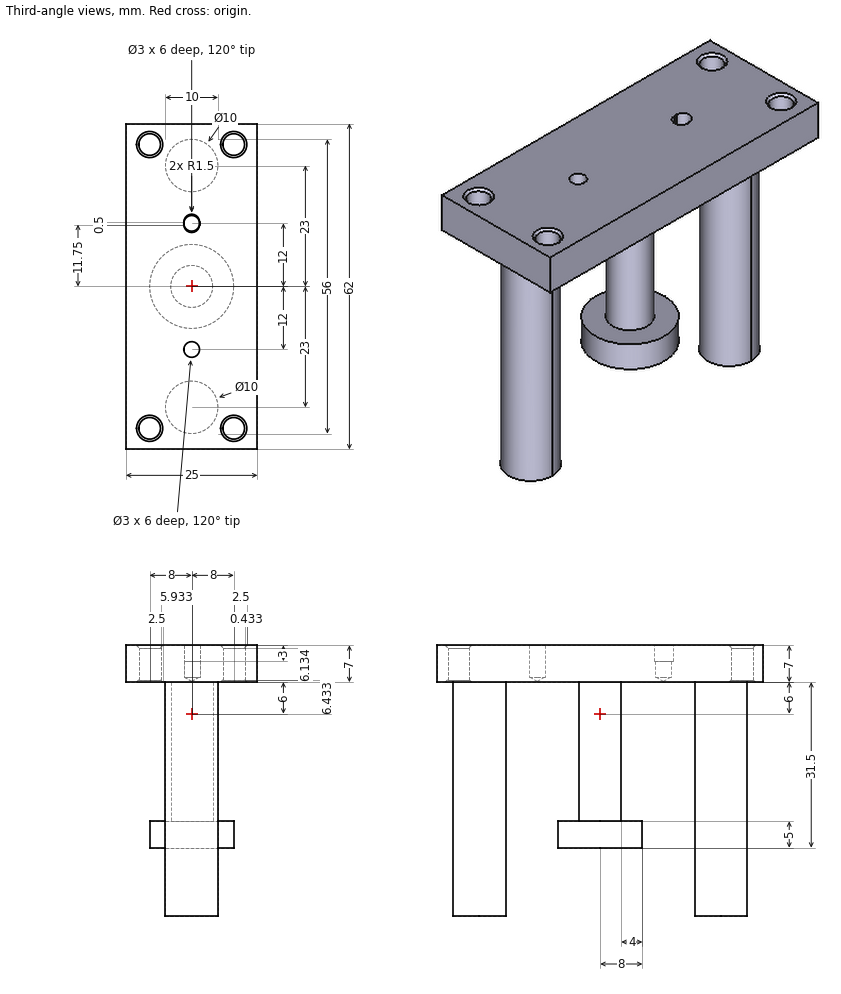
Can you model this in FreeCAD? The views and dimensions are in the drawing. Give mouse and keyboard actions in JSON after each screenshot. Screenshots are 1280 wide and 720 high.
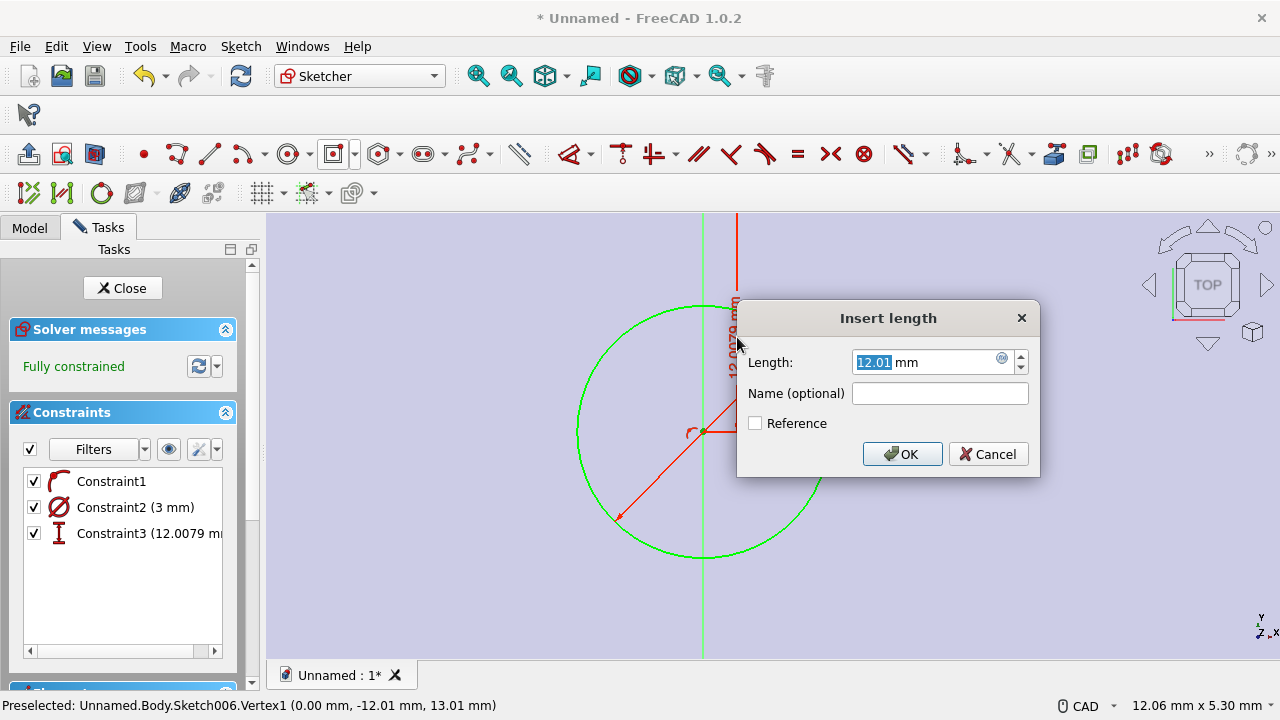
{"action": "type", "text": "12"}
{"action": "key", "text": "Return"}
{"action": "key", "text": "Escape"}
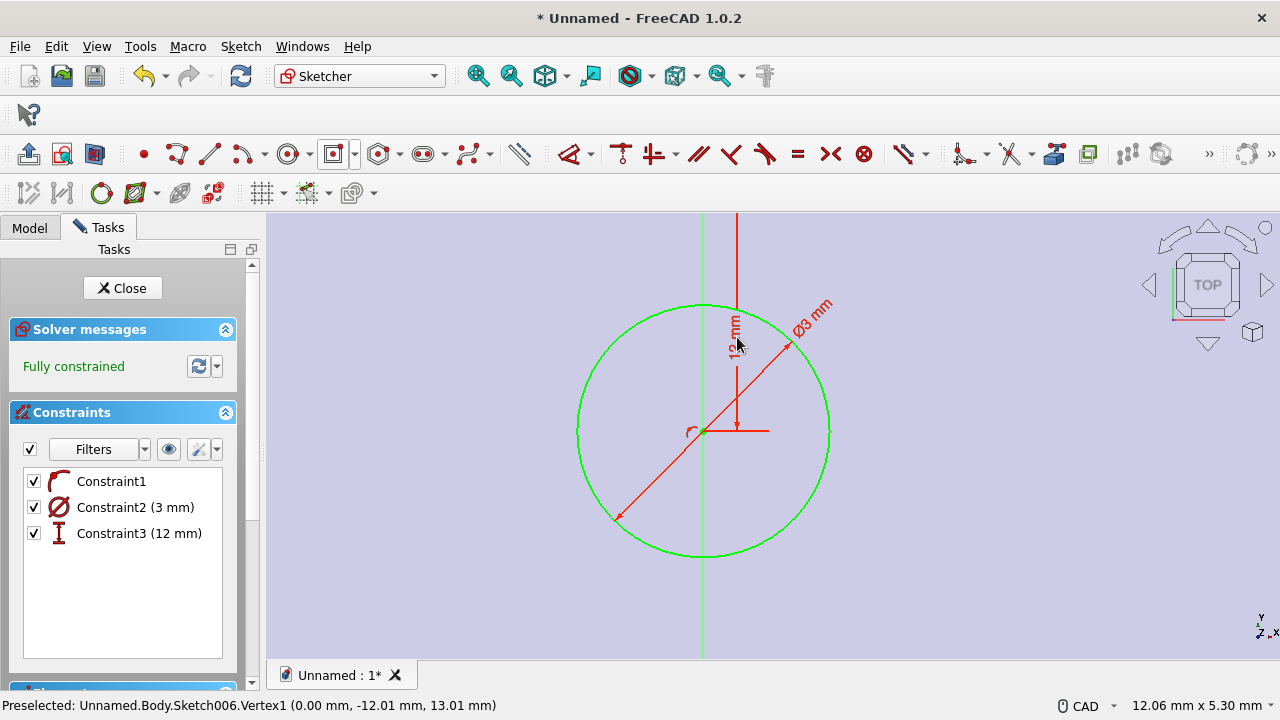
{"action": "left_click", "coordinate": [123, 288]}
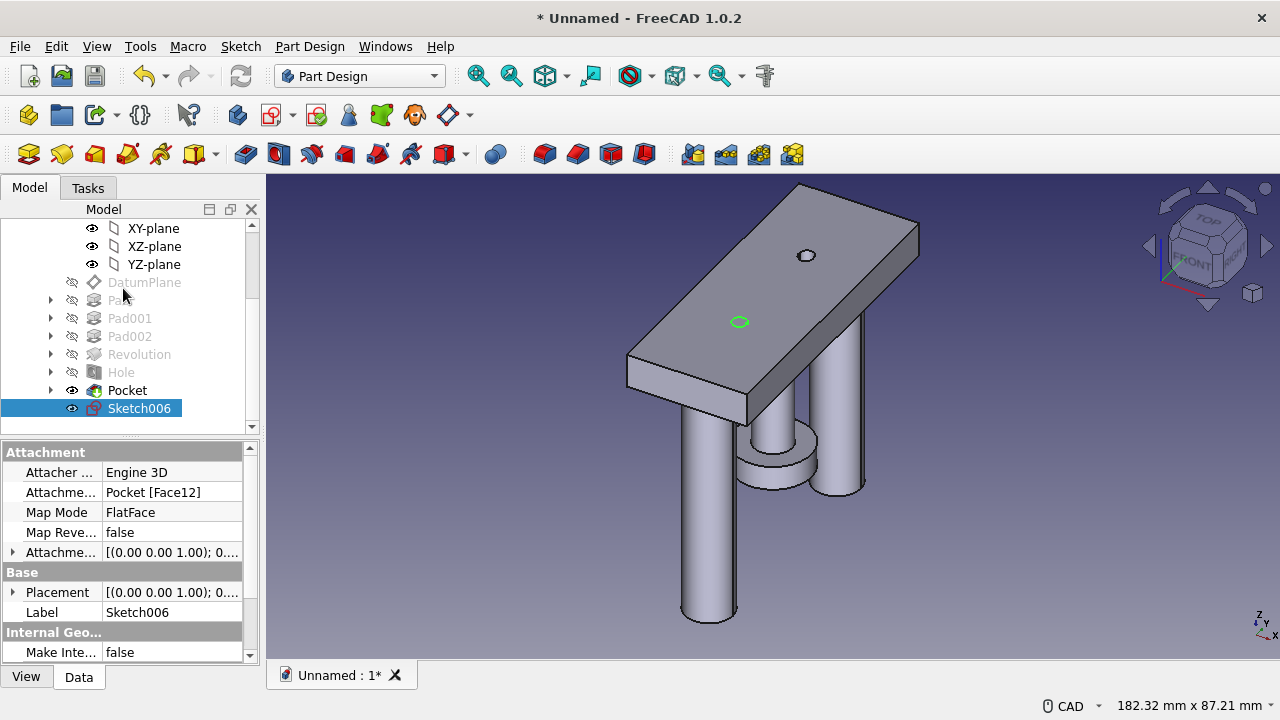
{"action": "left_click", "coordinate": [279, 154]}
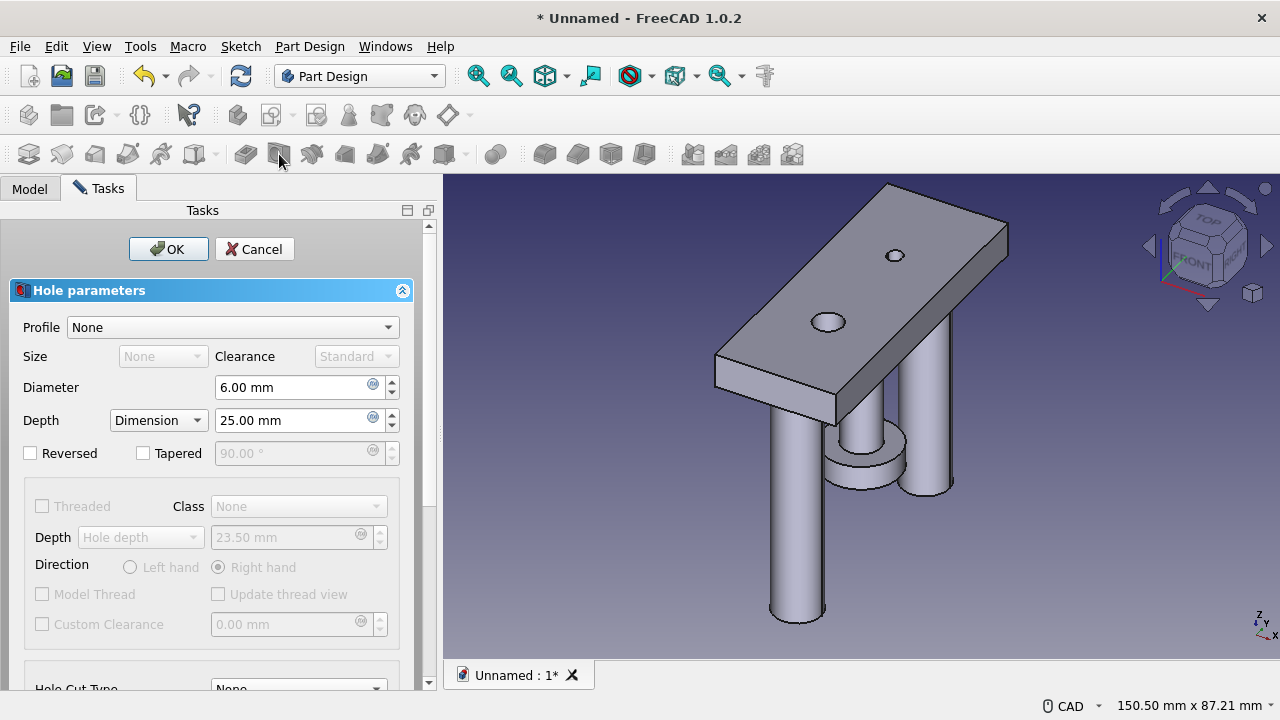
{"action": "triple_click", "coordinate": [300, 388]}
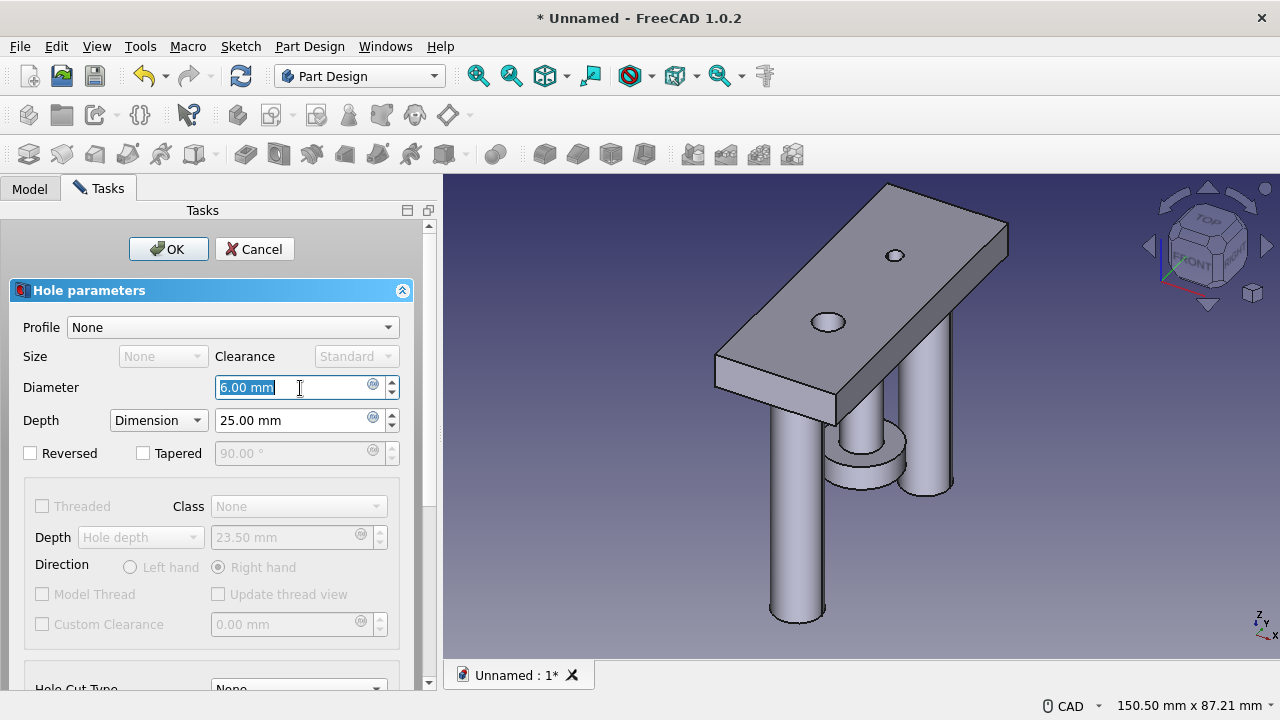
{"action": "type", "text": "3"}
{"action": "key", "text": "Tab"}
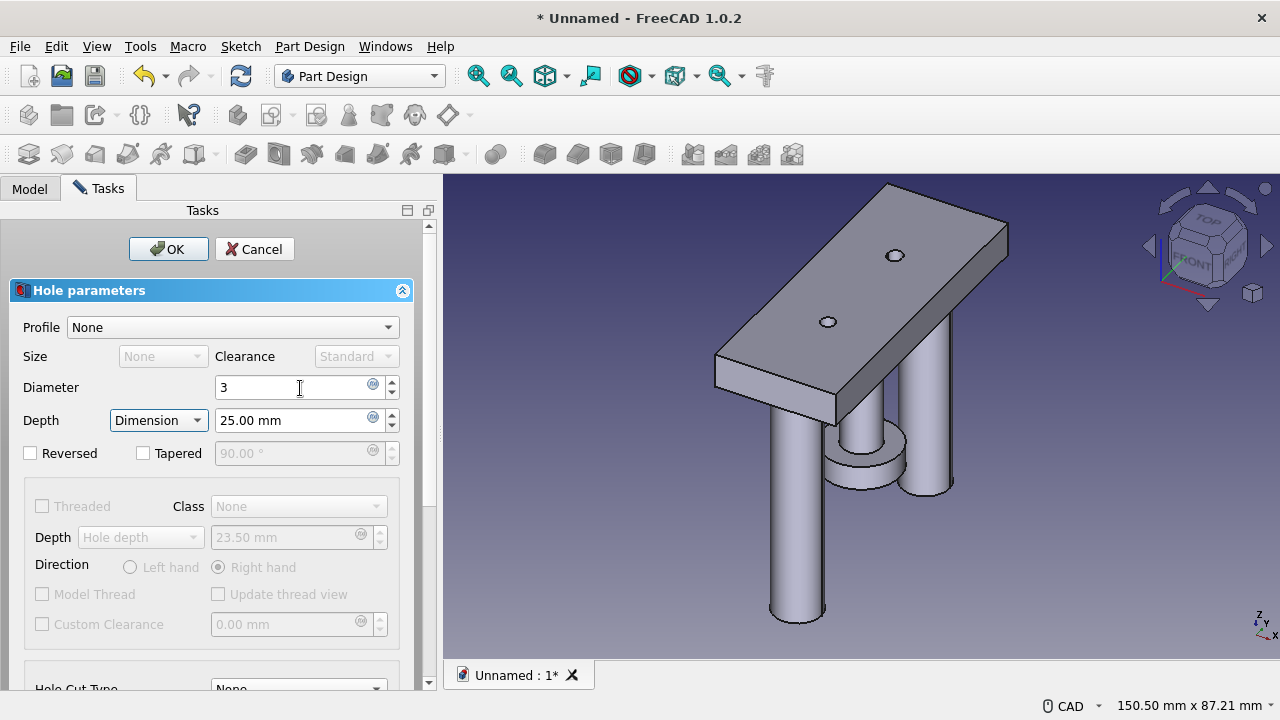
{"action": "triple_click", "coordinate": [300, 420]}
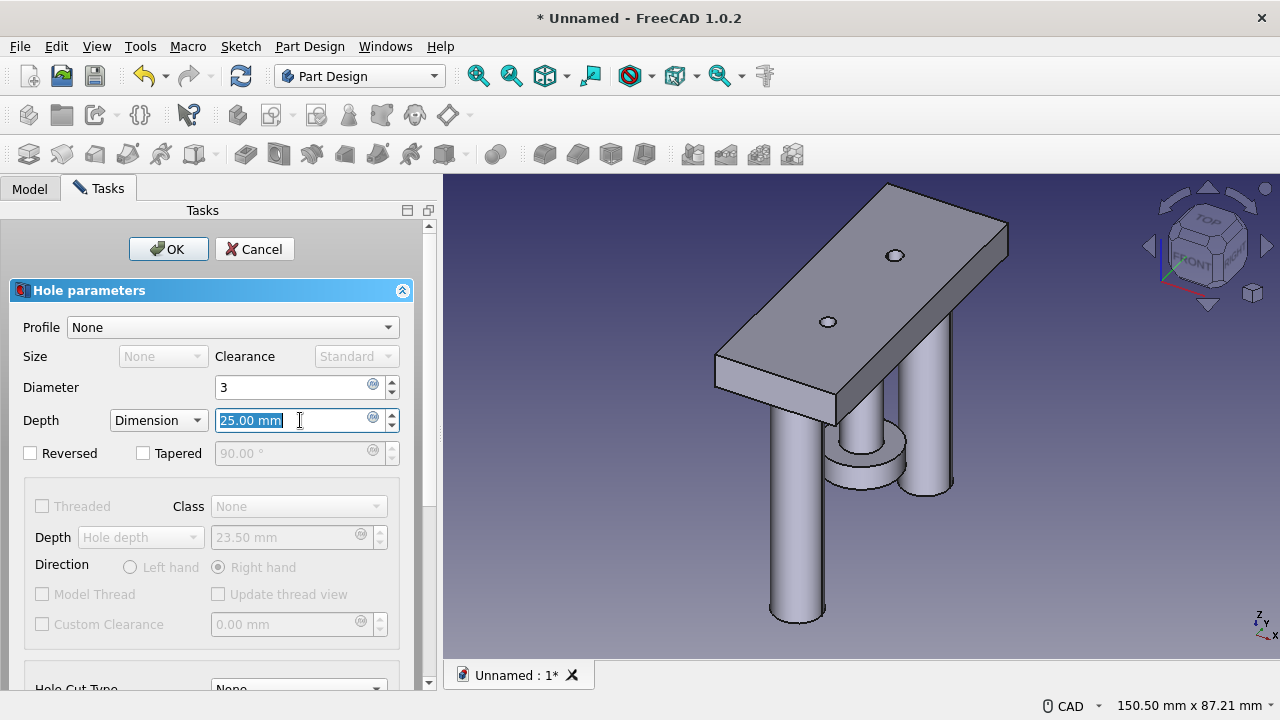
{"action": "type", "text": "6"}
{"action": "key", "text": "Tab"}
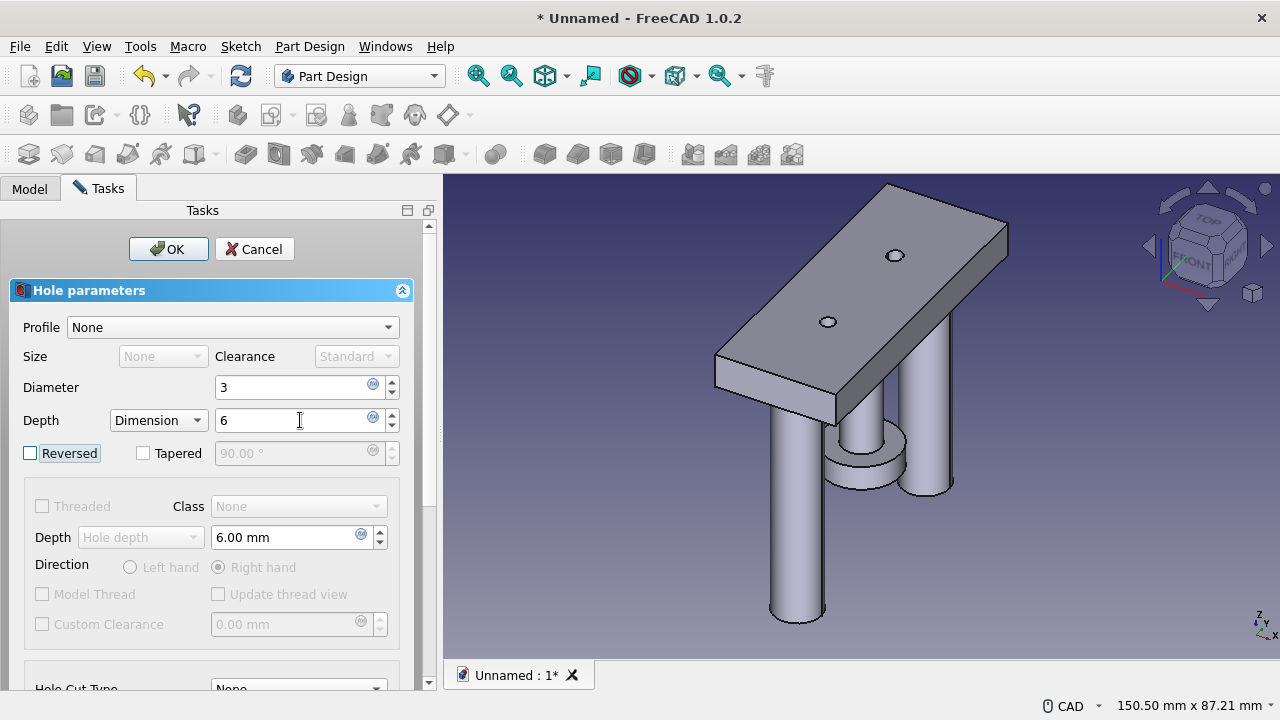
{"action": "scroll", "coordinate": [429, 455], "scroll_direction": "down", "scroll_amount": 5}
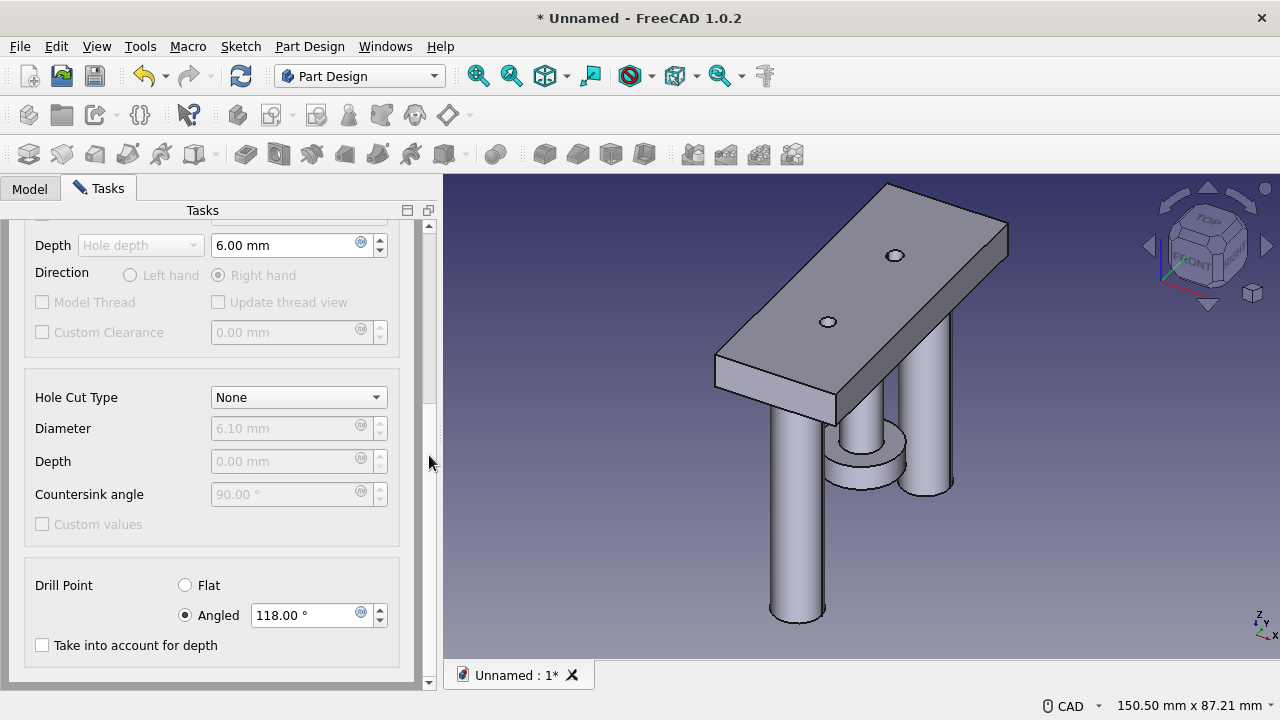
{"action": "triple_click", "coordinate": [312, 616]}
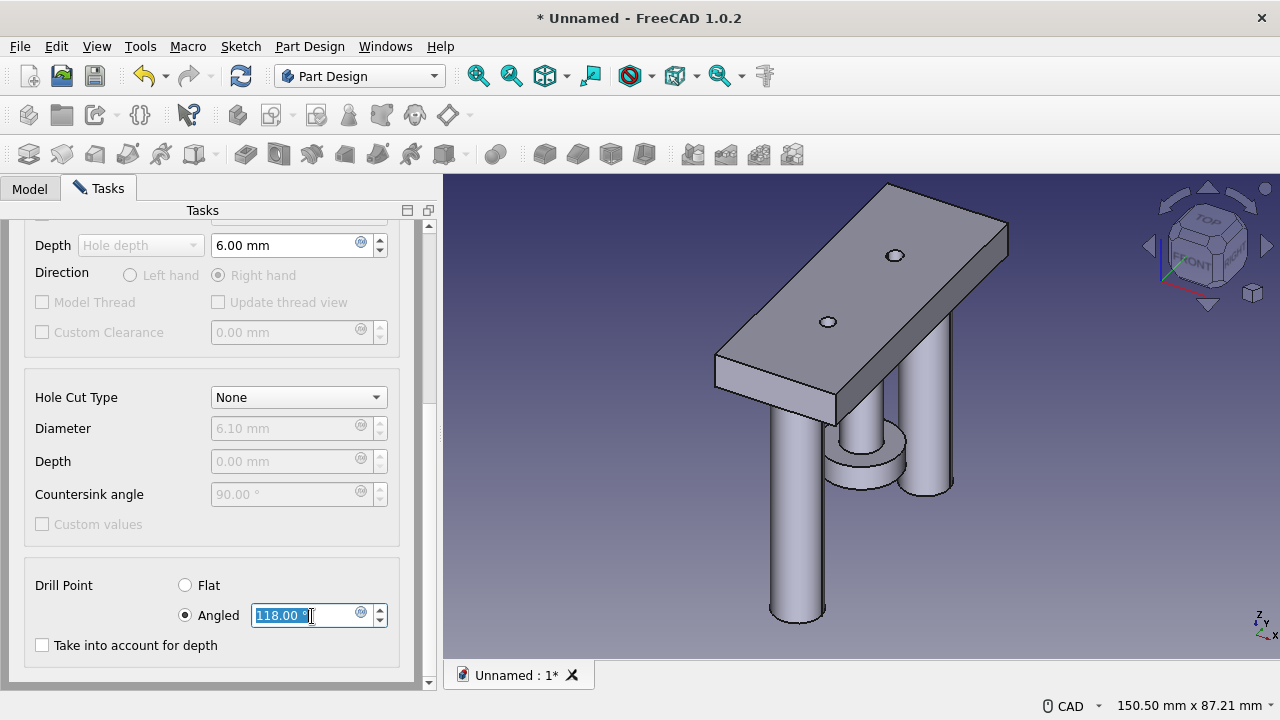
{"action": "type", "text": "120"}
{"action": "key", "text": "Tab"}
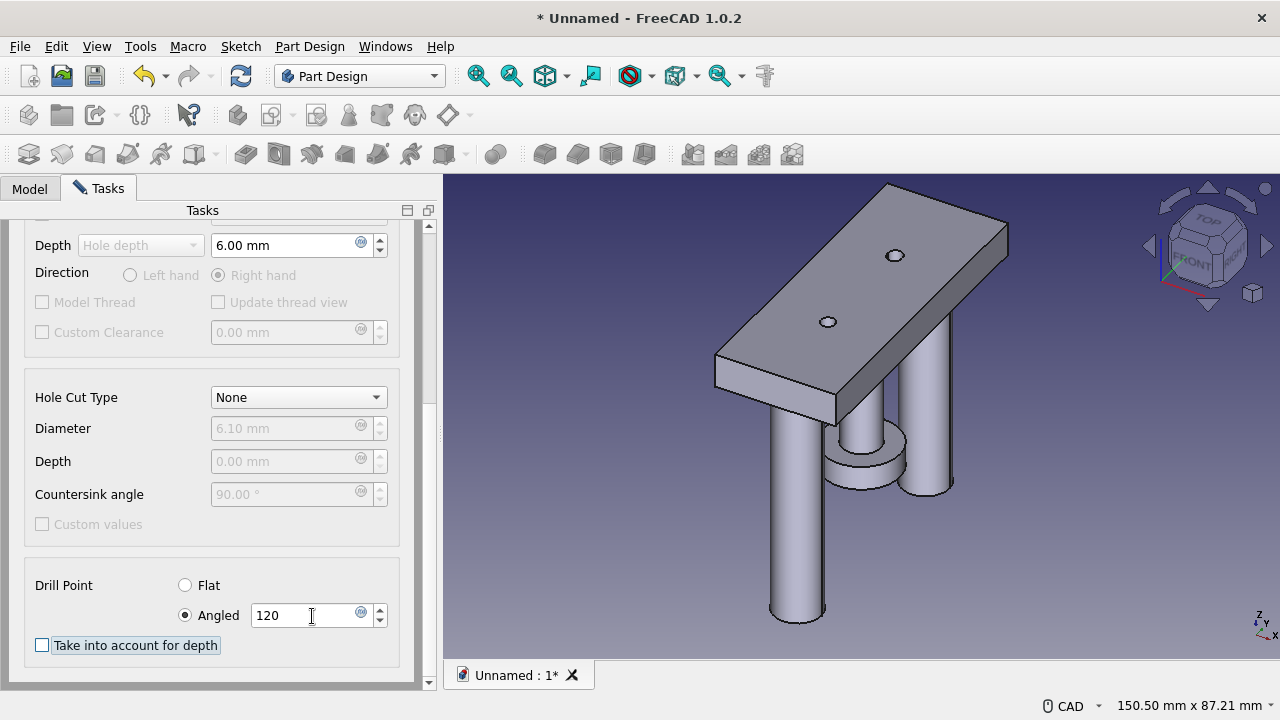
{"action": "scroll", "coordinate": [429, 455], "scroll_direction": "up", "scroll_amount": 6}